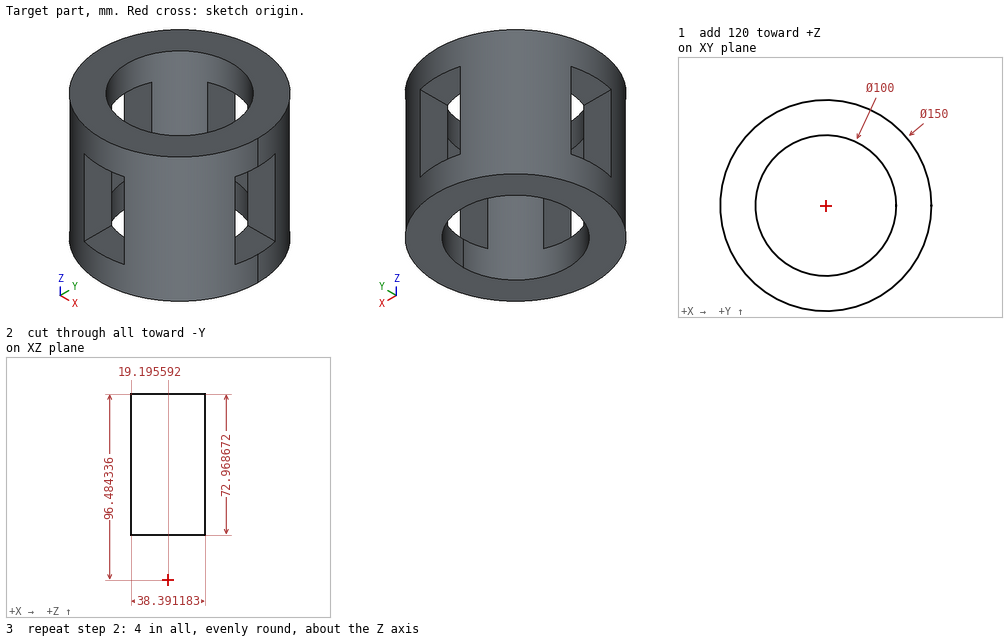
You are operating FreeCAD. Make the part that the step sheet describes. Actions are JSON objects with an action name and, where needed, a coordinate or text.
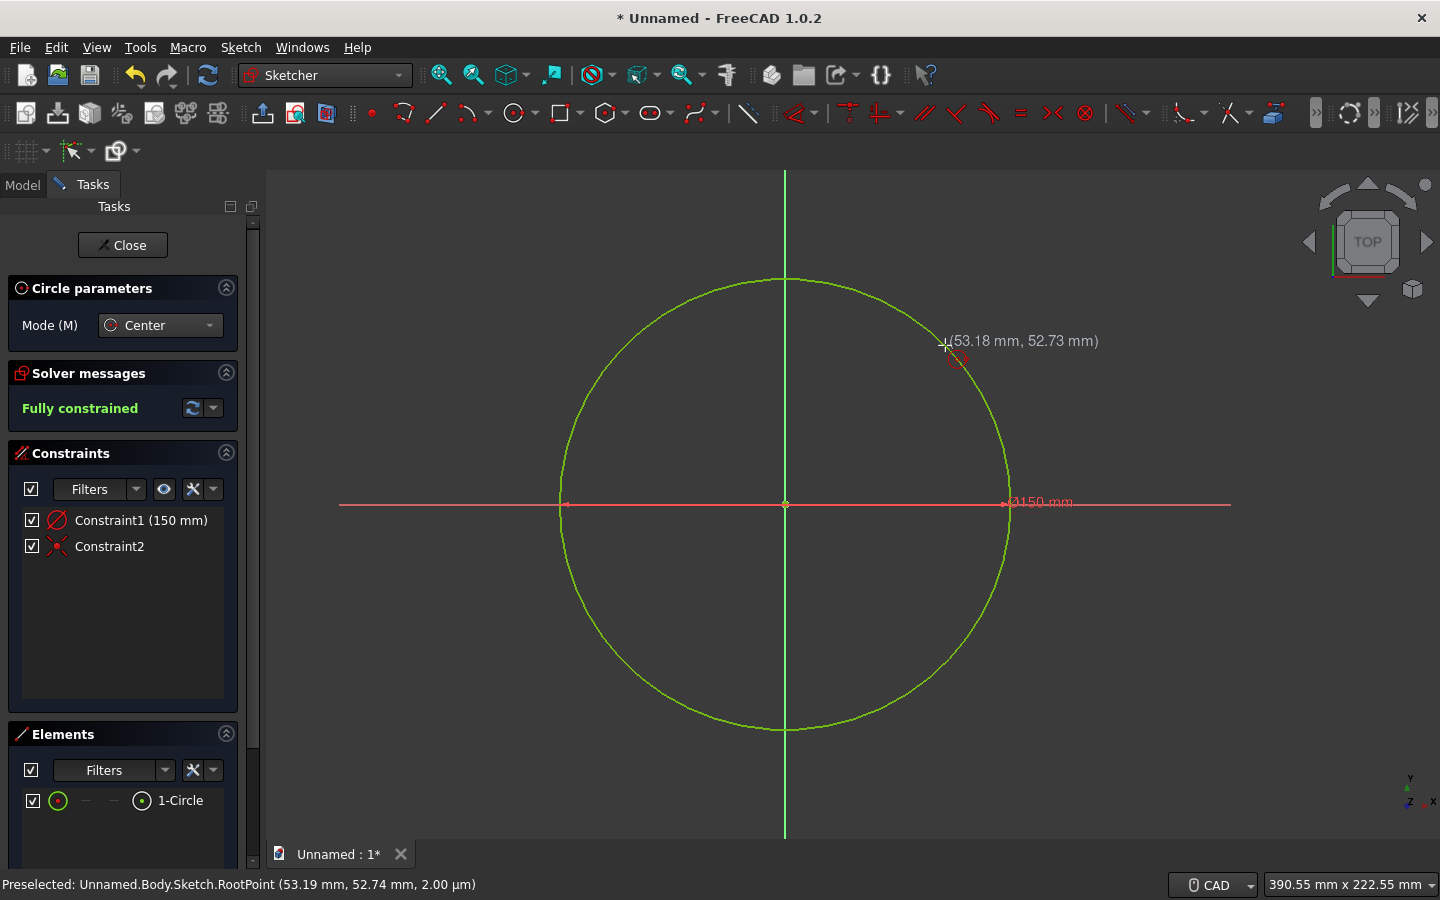
{"action": "left_click", "coordinate": [785, 504]}
{"action": "mouse_move", "coordinate": [891, 398]}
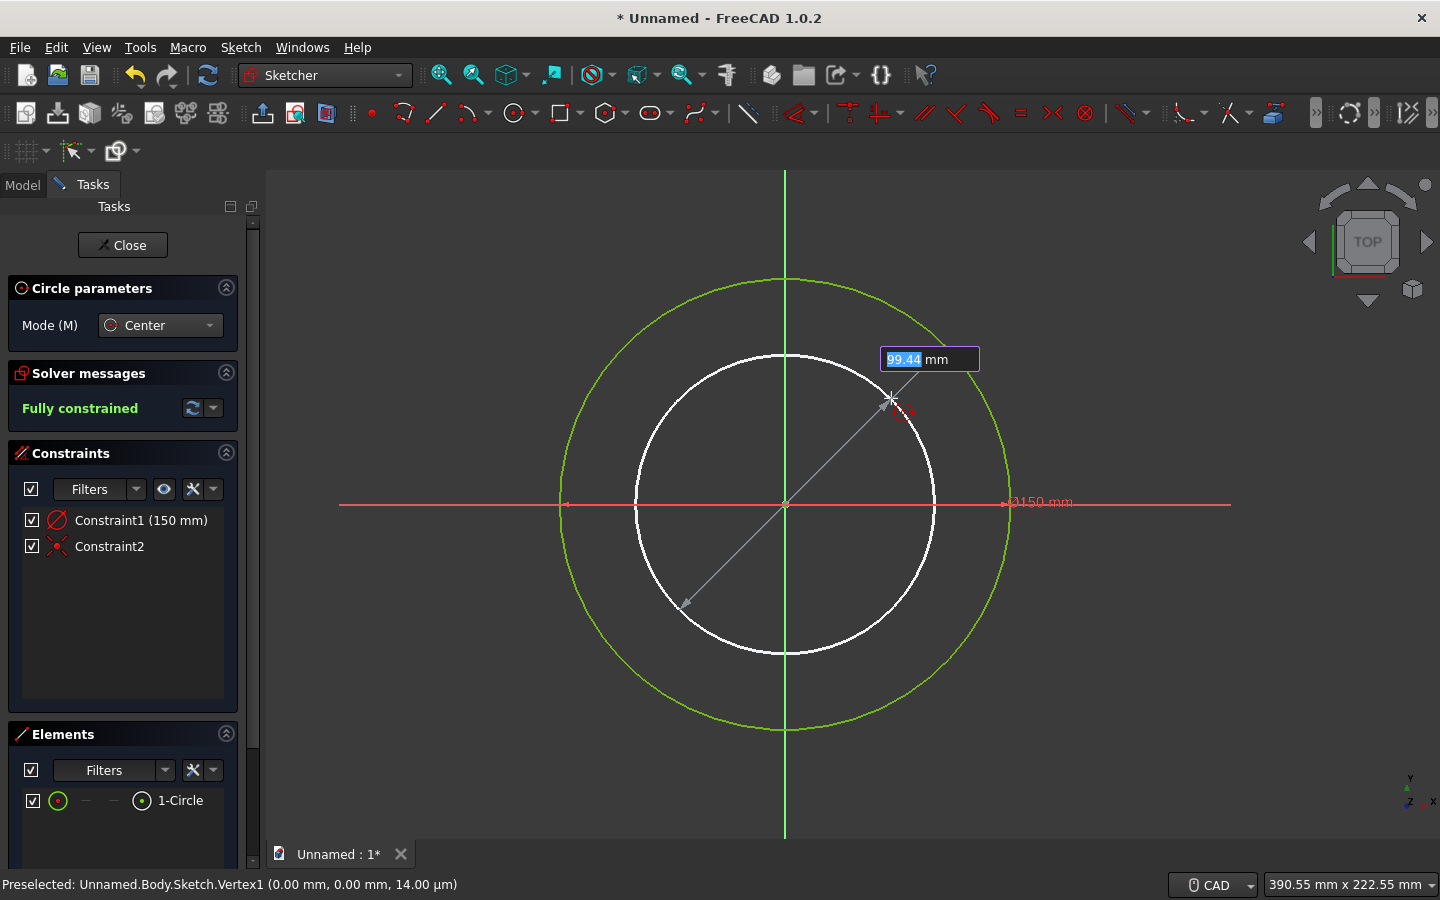
{"action": "type", "text": "100"}
{"action": "key", "text": "Return"}
{"action": "key", "text": "Escape"}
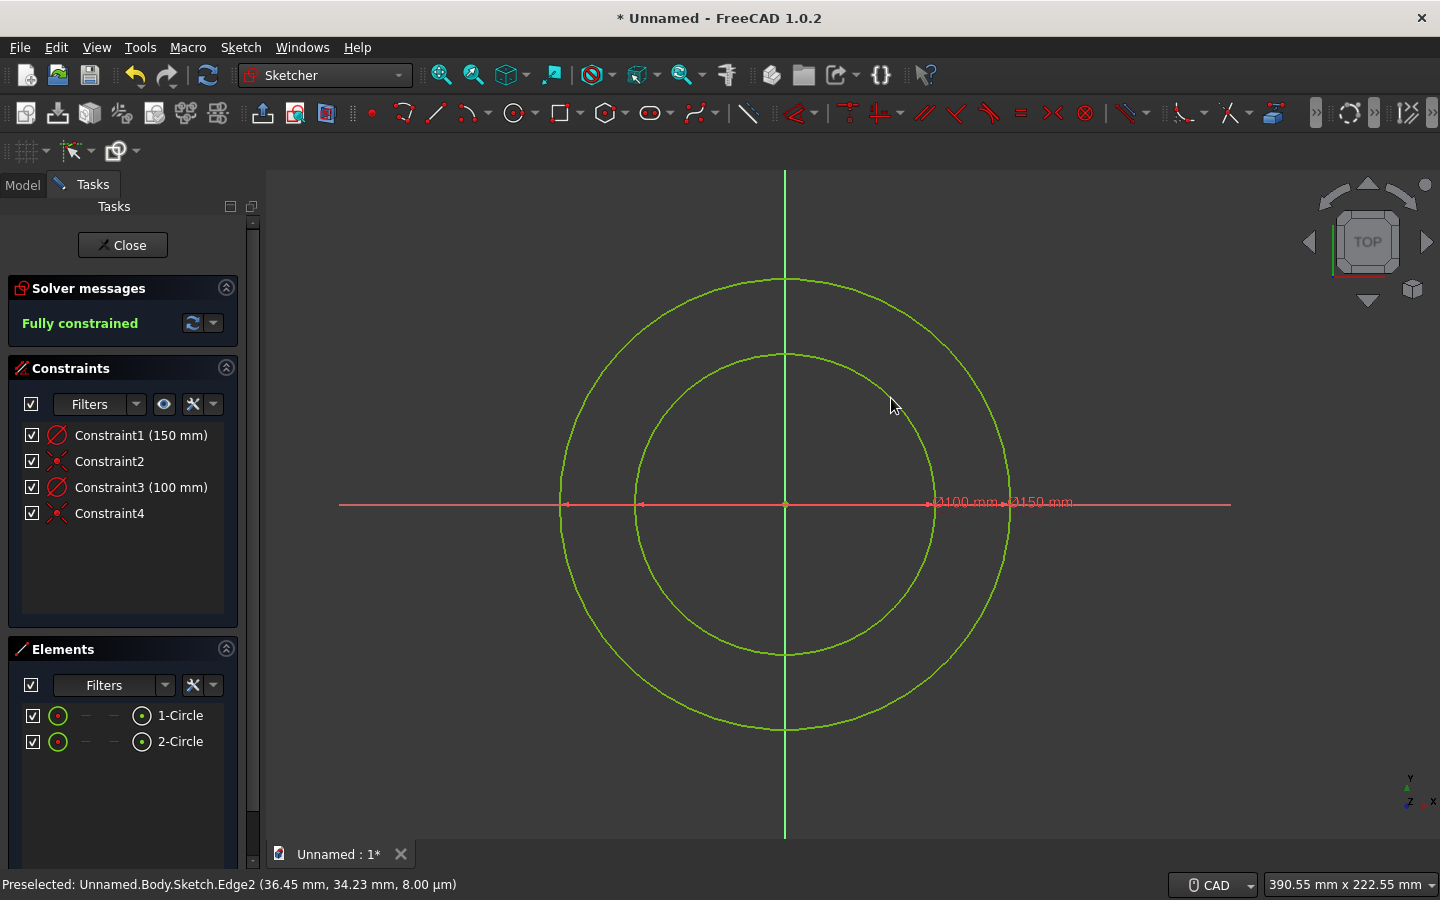
{"action": "left_click", "coordinate": [123, 245]}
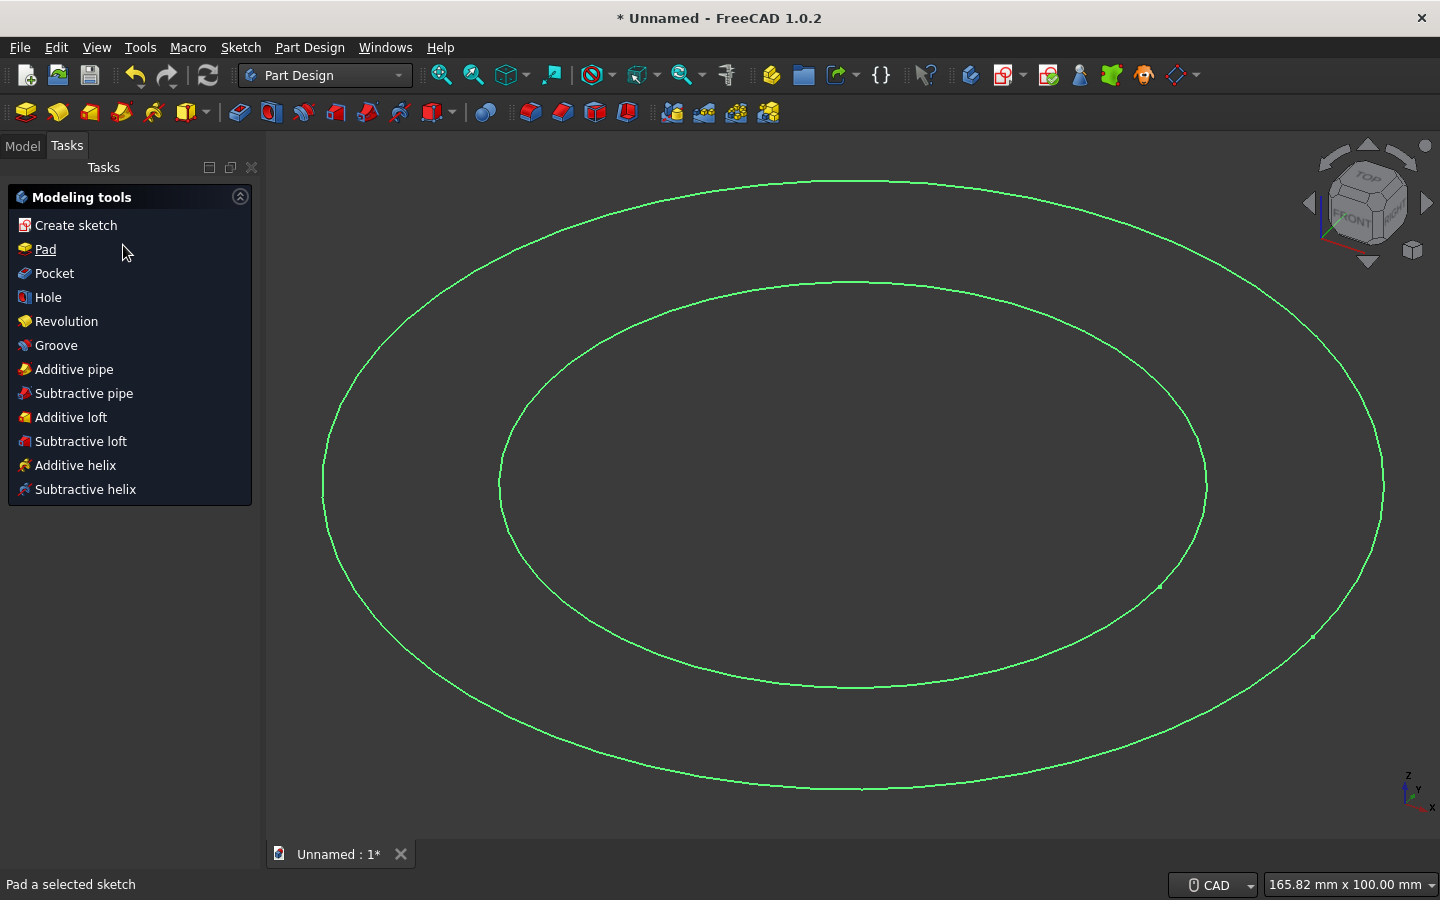
{"action": "left_click", "coordinate": [26, 112]}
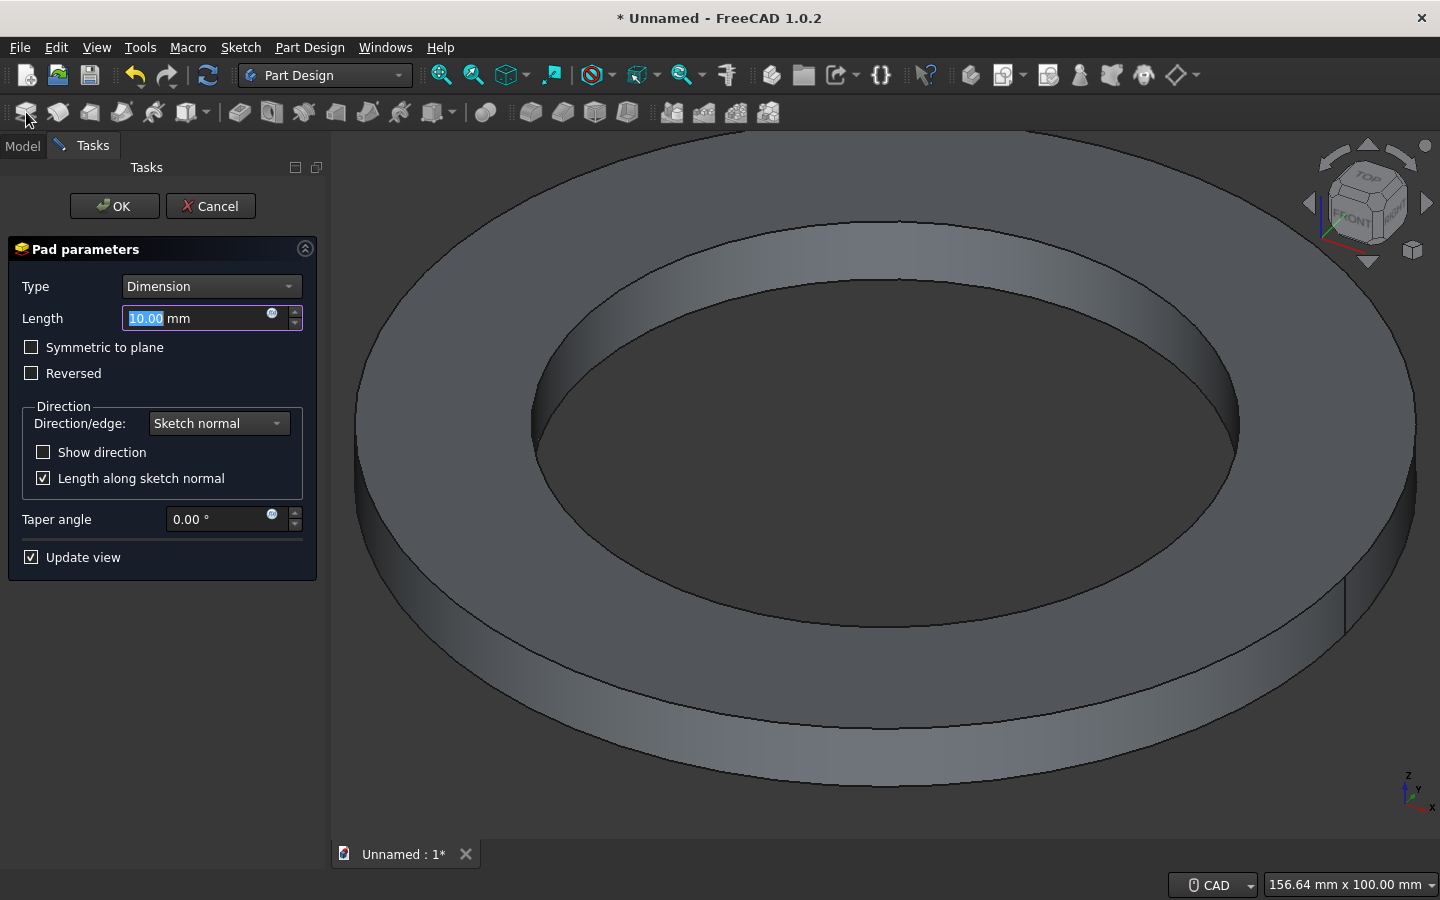
{"action": "type", "text": "120"}
{"action": "key", "text": "Tab"}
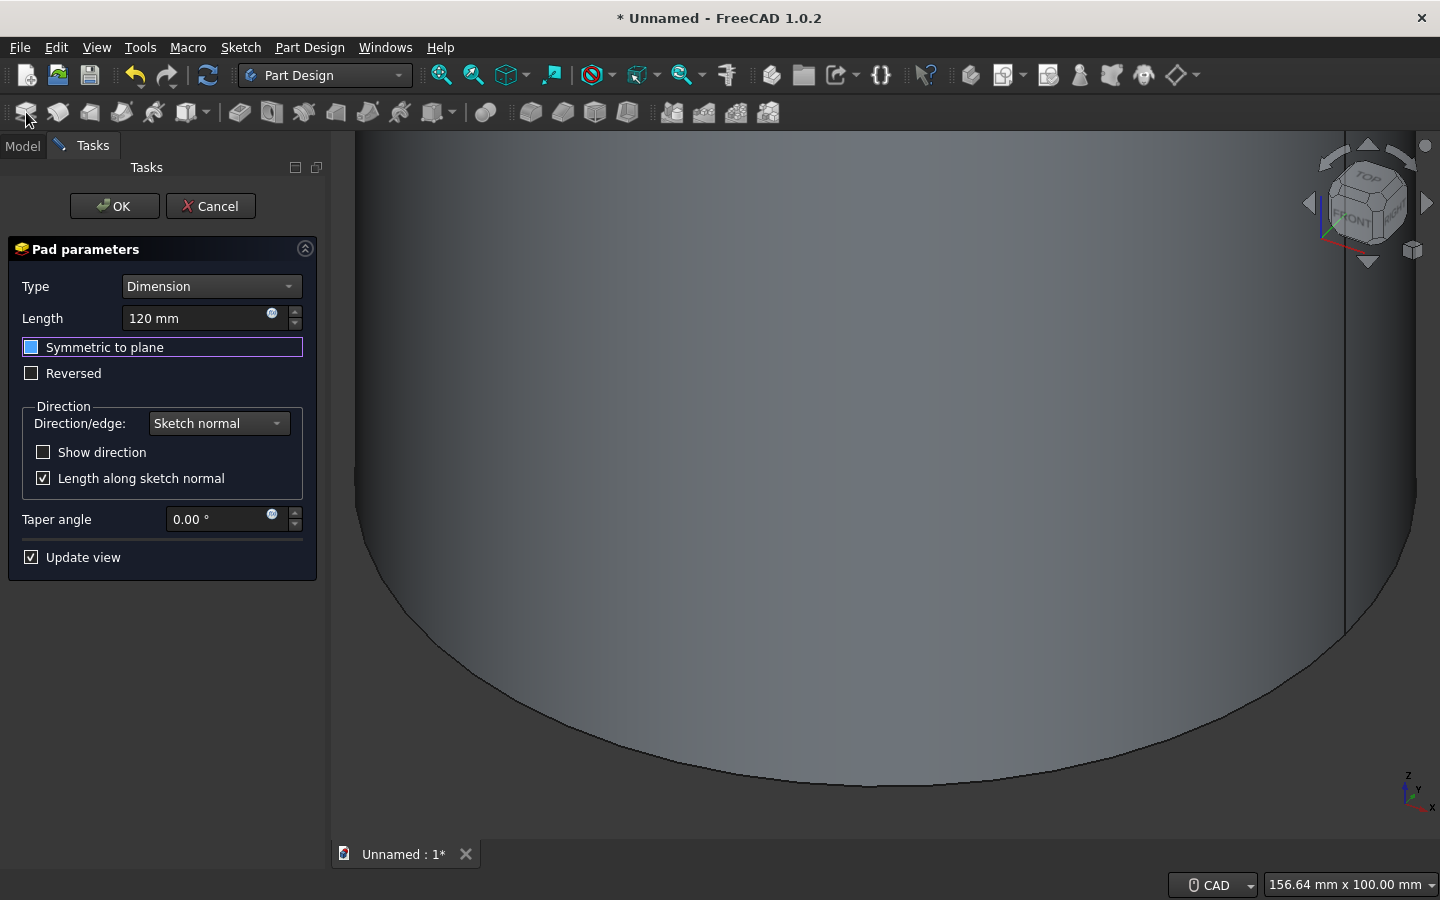
{"action": "left_click", "coordinate": [115, 206]}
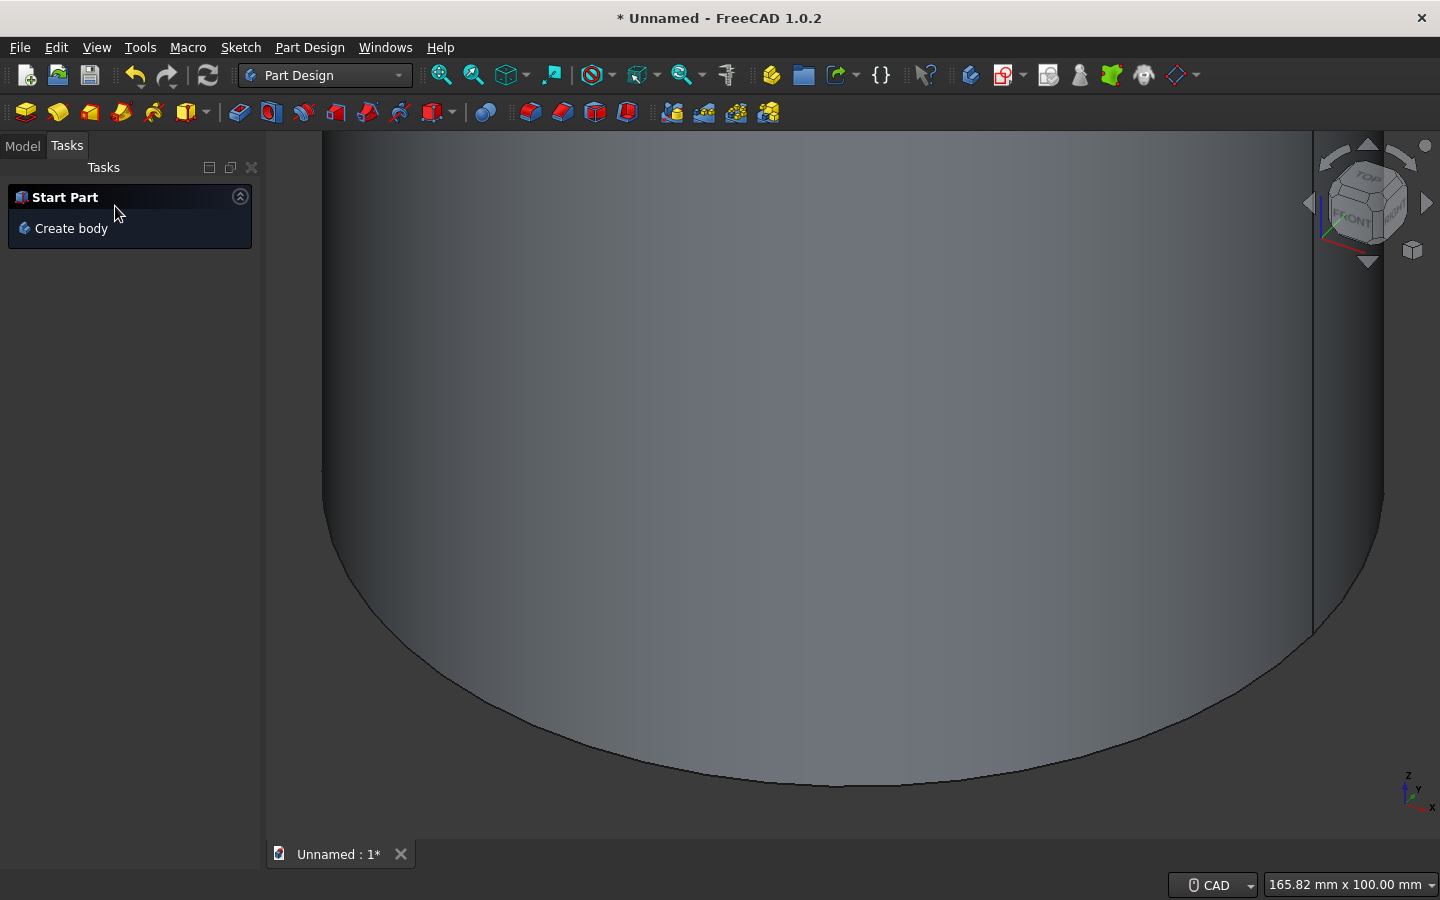
{"action": "left_click", "coordinate": [442, 76]}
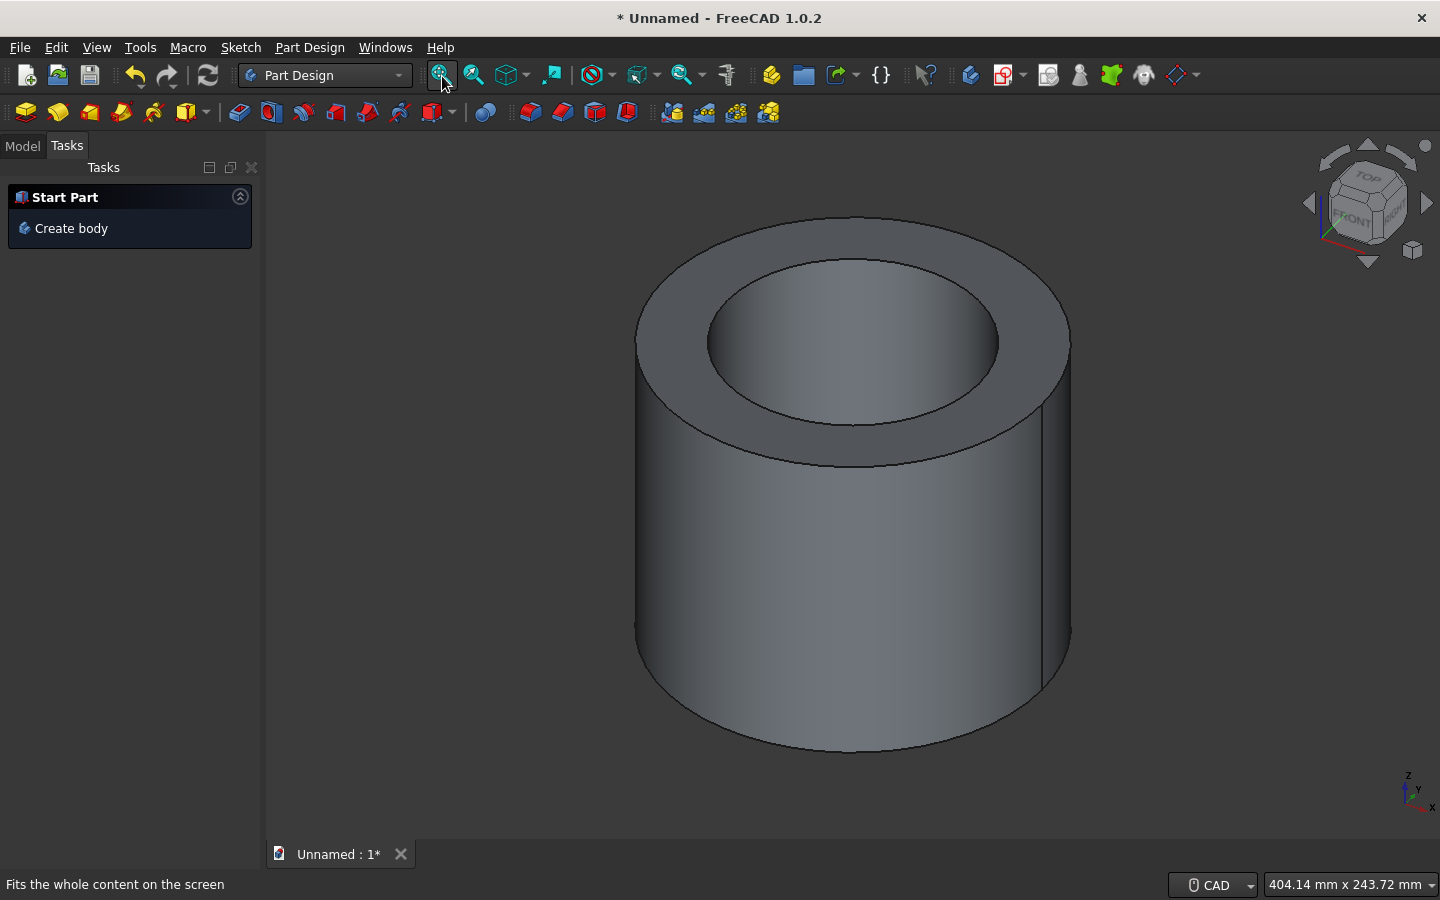
{"action": "left_click", "coordinate": [1004, 76]}